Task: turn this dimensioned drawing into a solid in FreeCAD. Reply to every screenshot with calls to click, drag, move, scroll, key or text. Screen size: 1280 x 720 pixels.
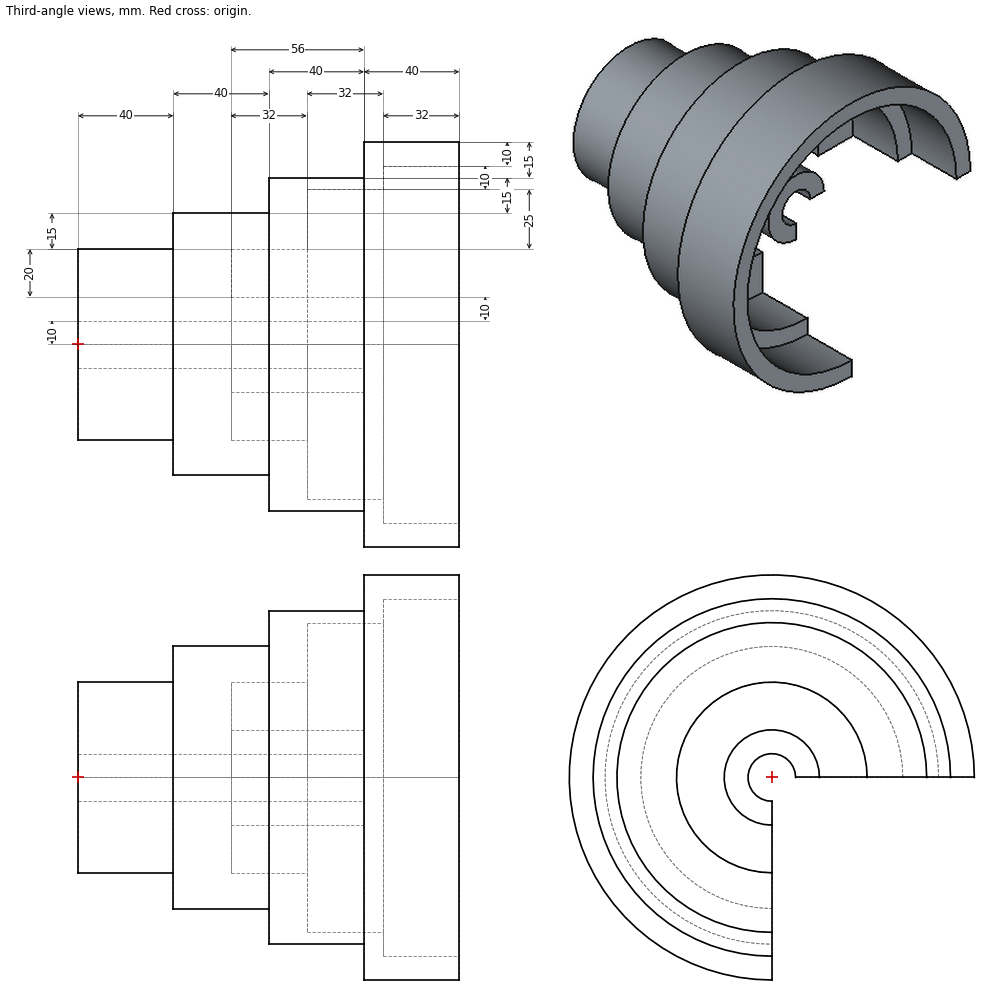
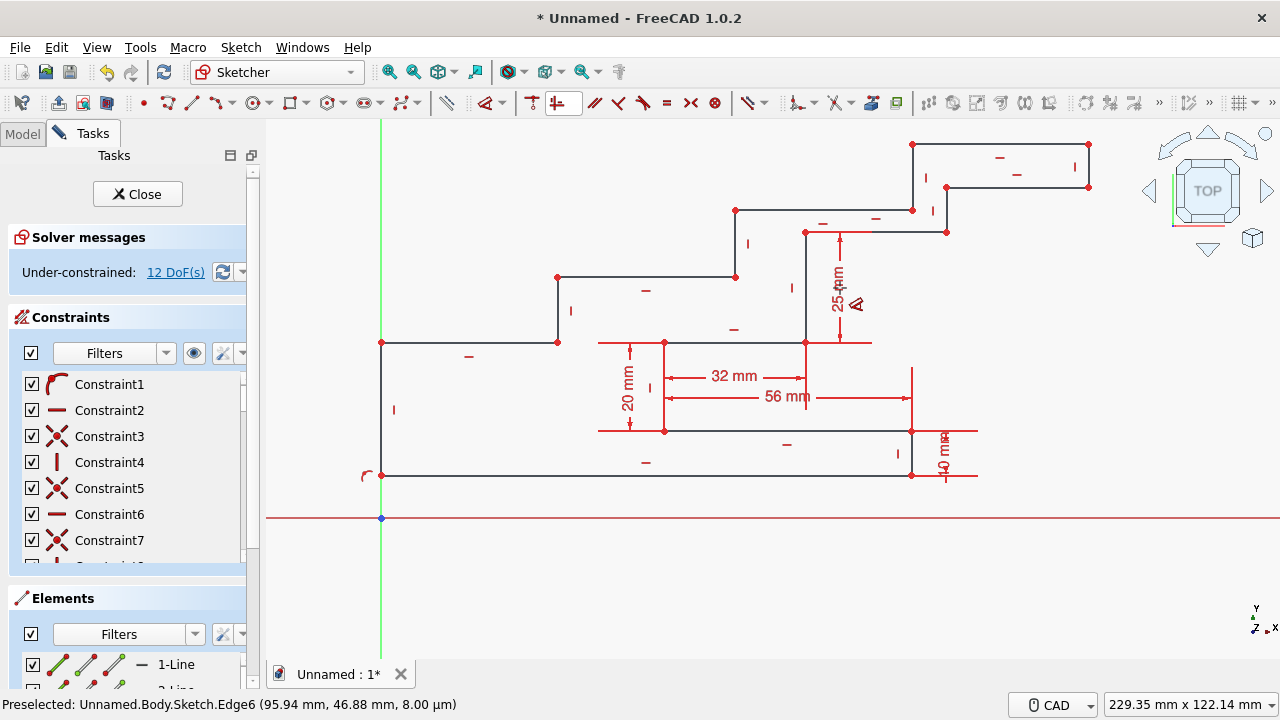
click(848, 232)
click(926, 198)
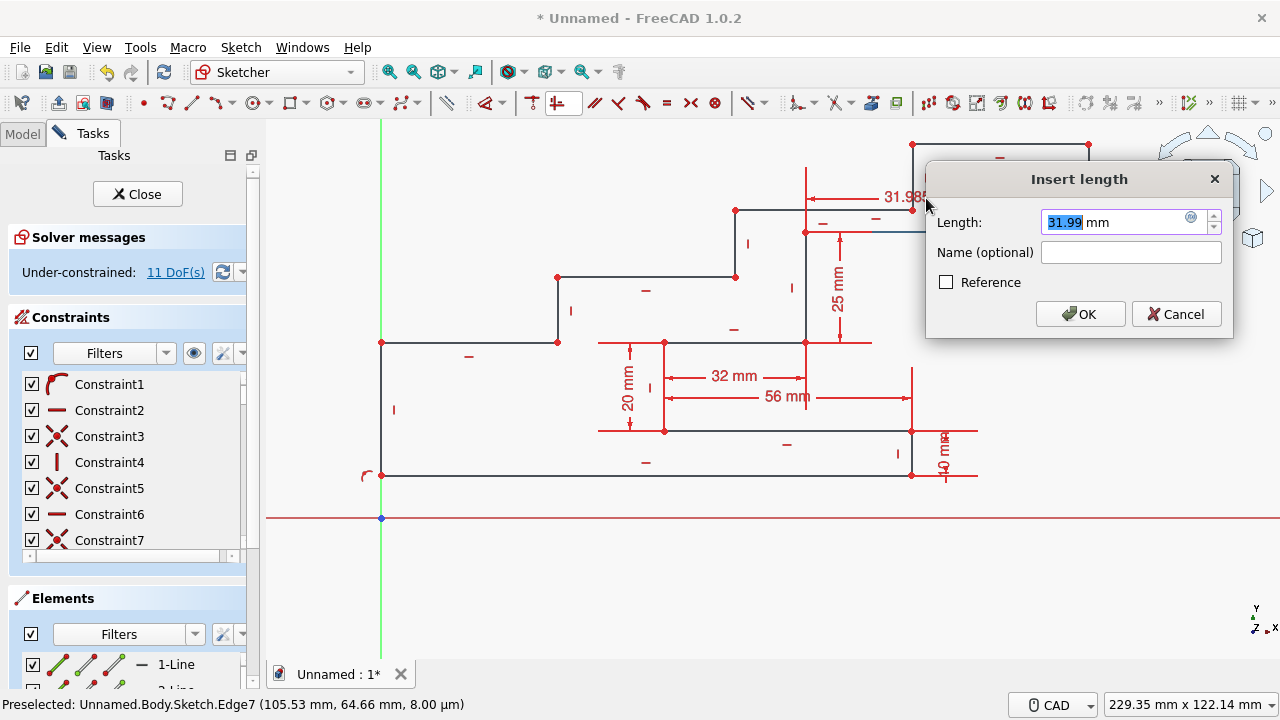
text(32)
key(Return)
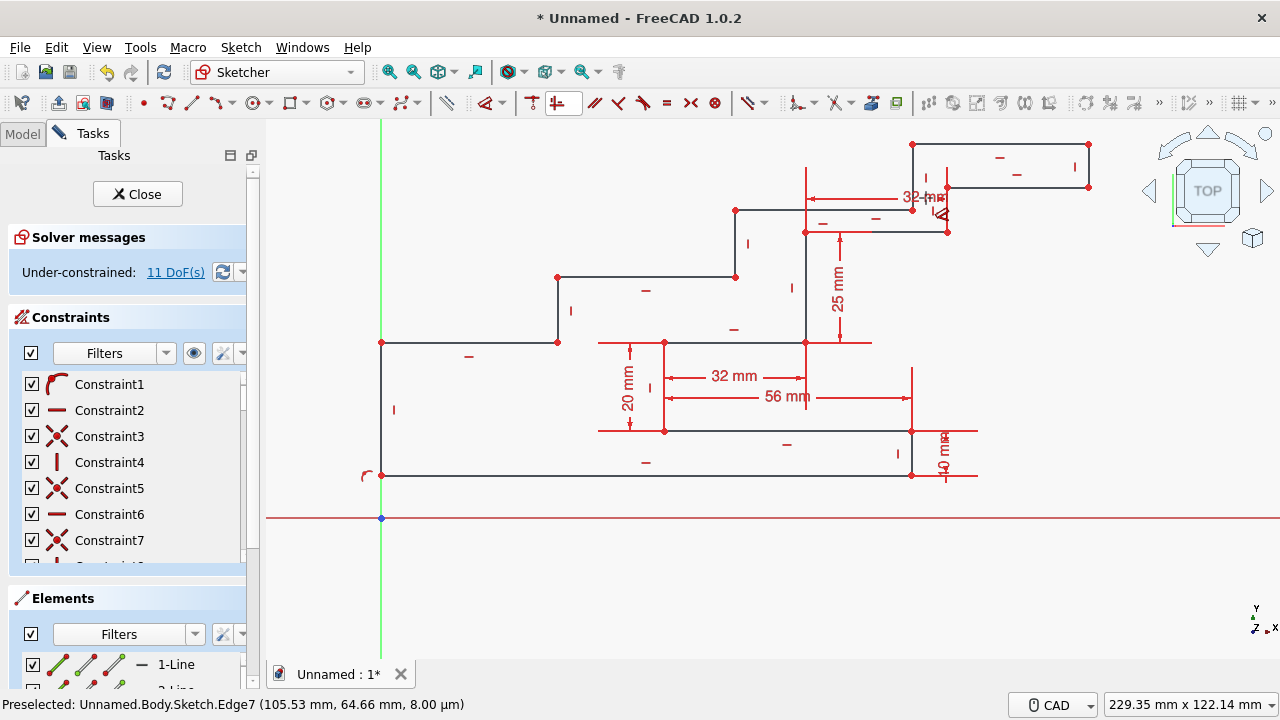
click(947, 219)
click(981, 220)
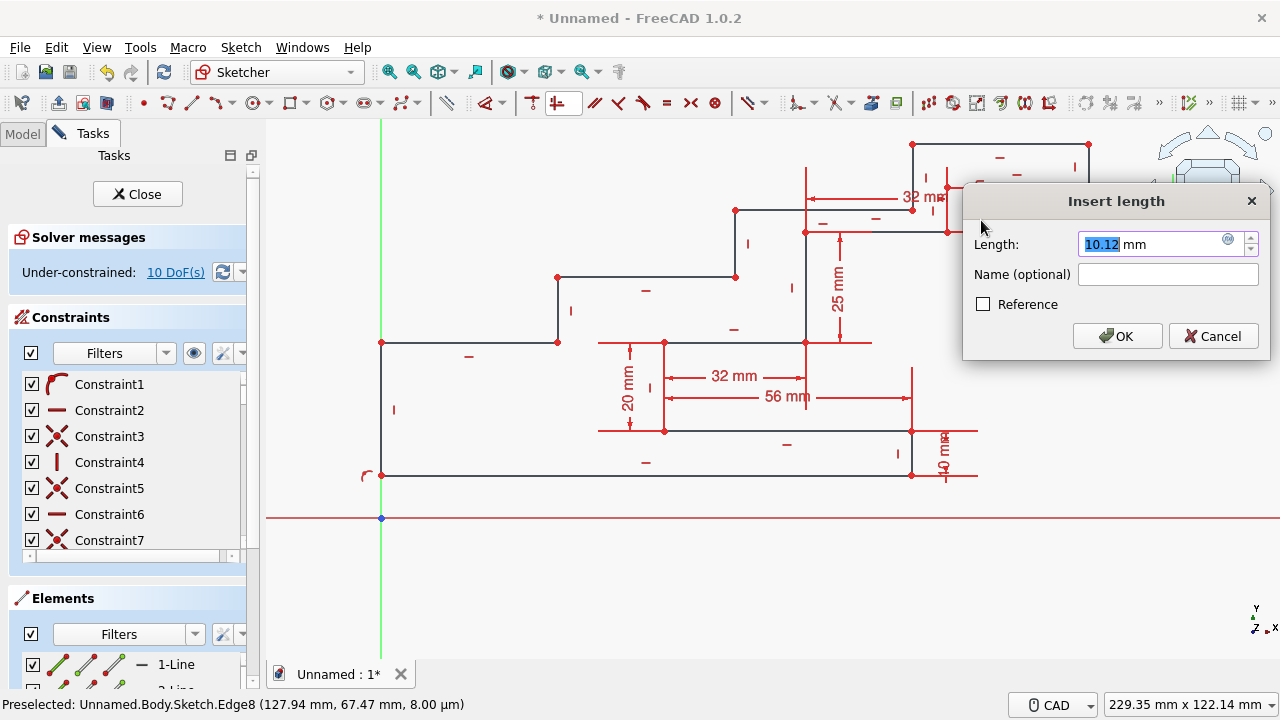
text(10)
key(Return)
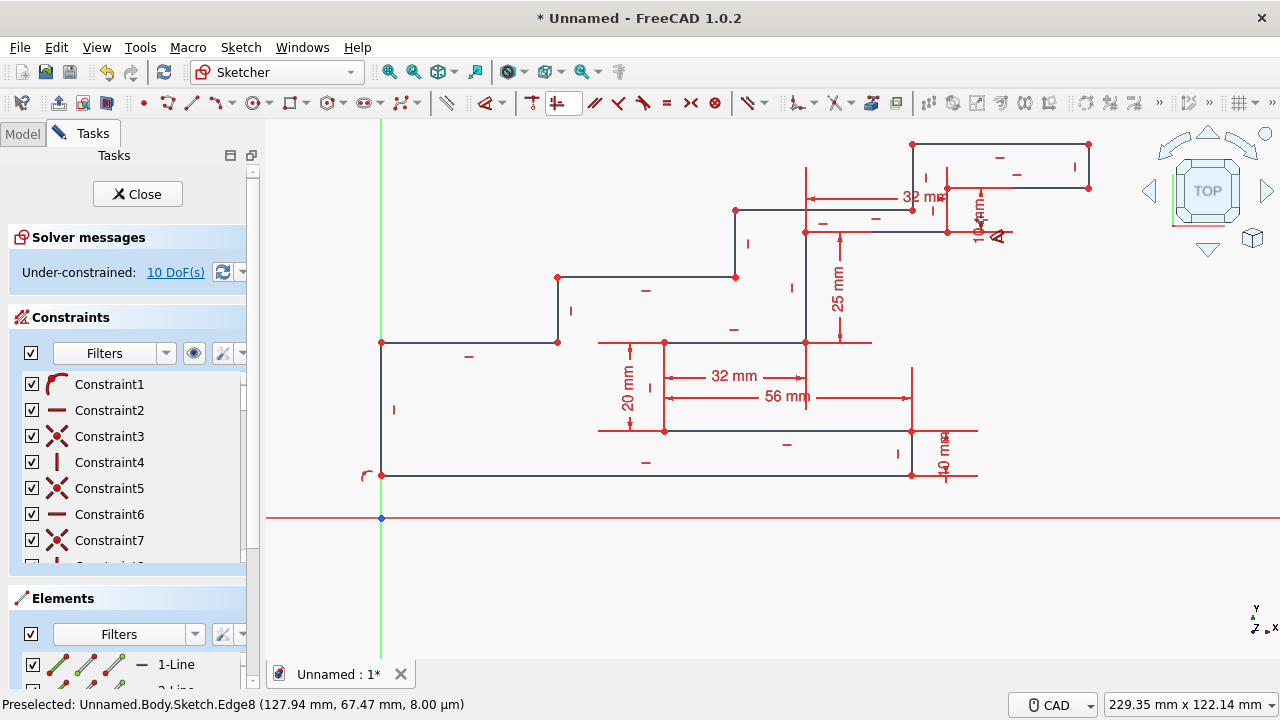
click(990, 188)
click(1067, 222)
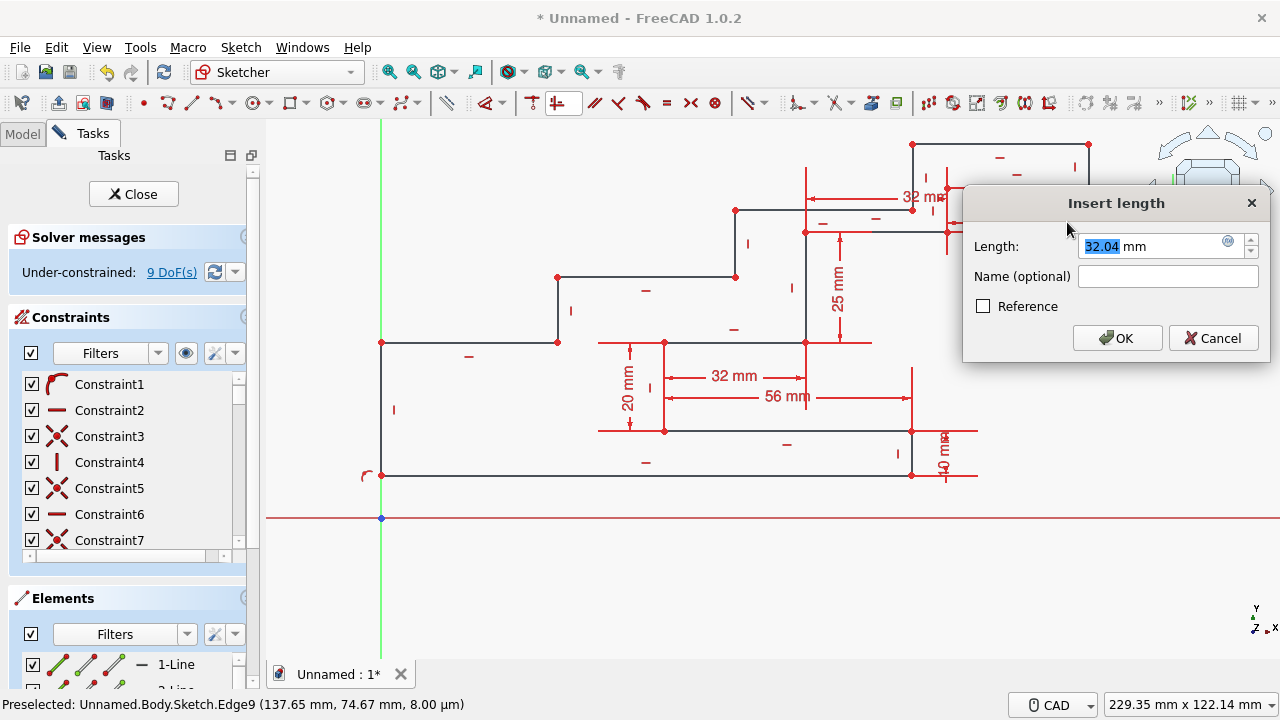
text(32)
key(Return)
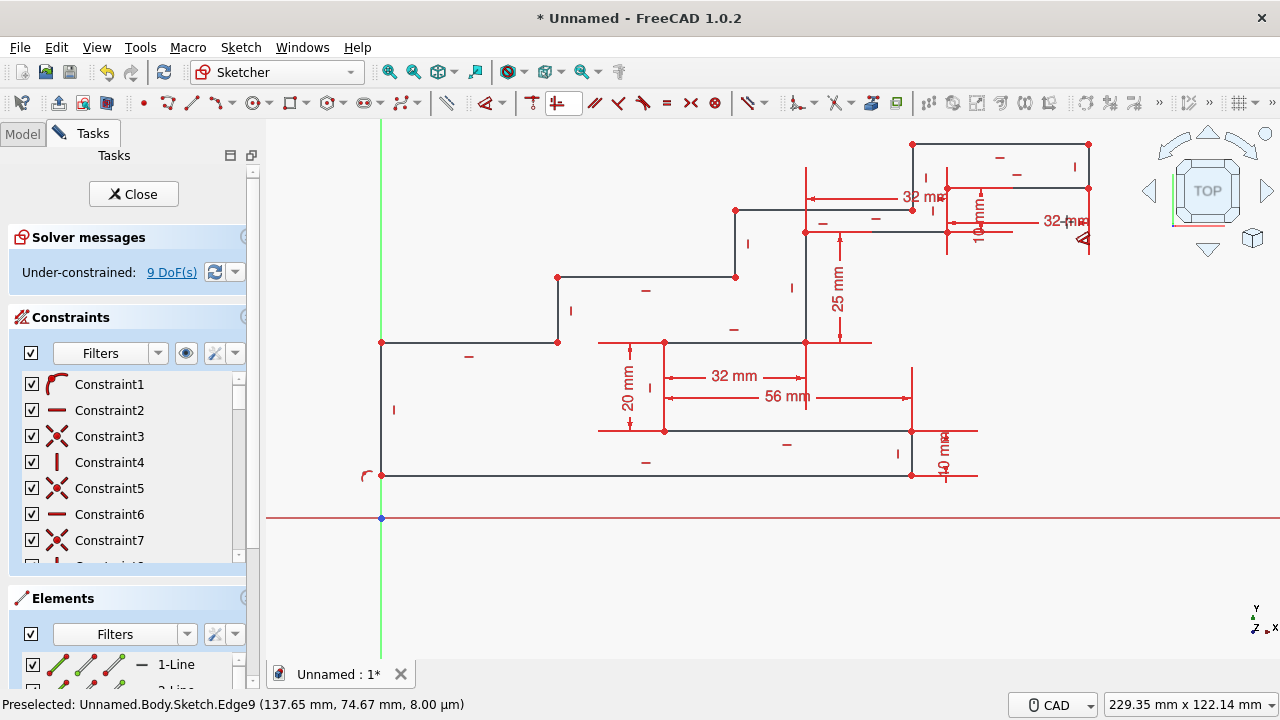
click(1089, 175)
click(1055, 168)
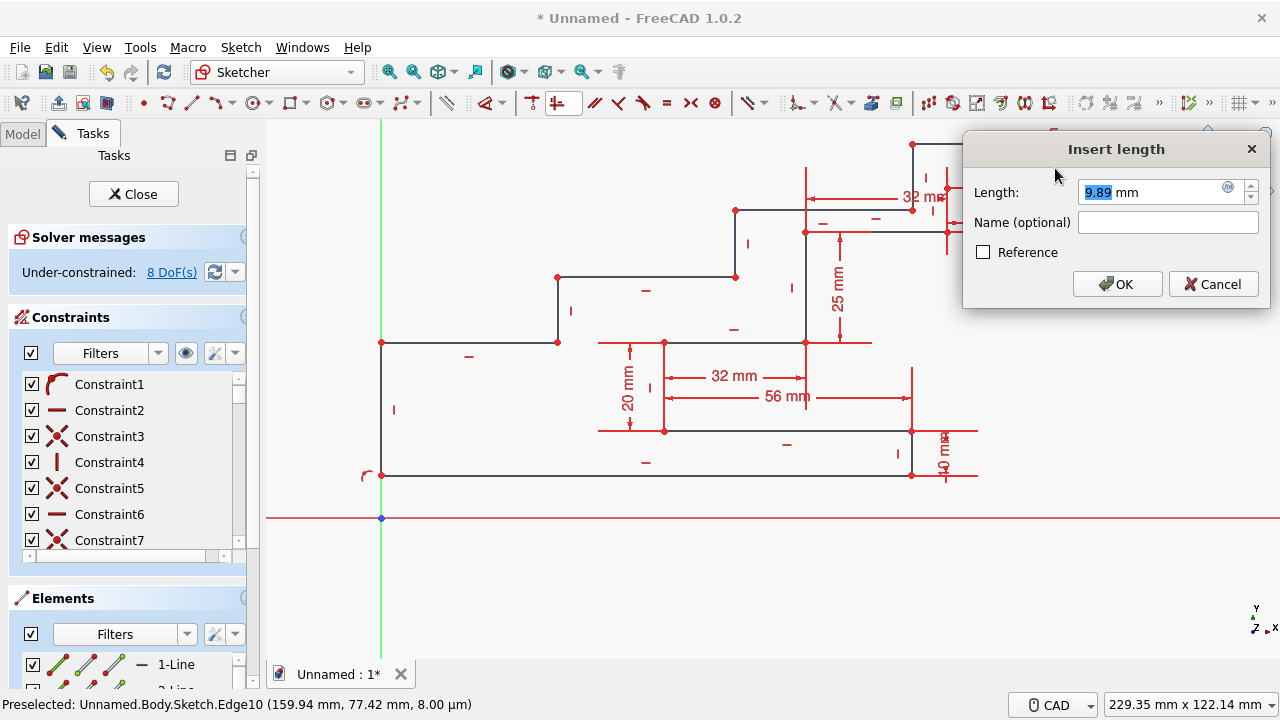
text(10)
key(Return)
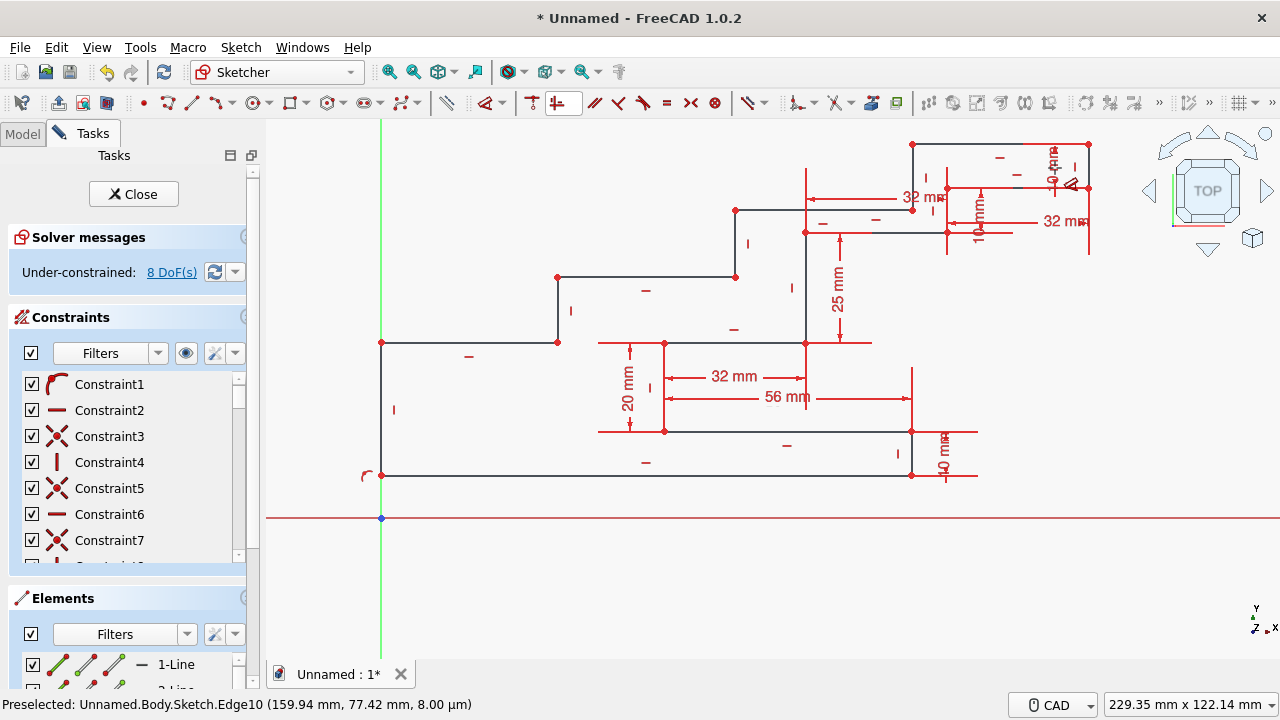
scroll(566, 631, down, 1)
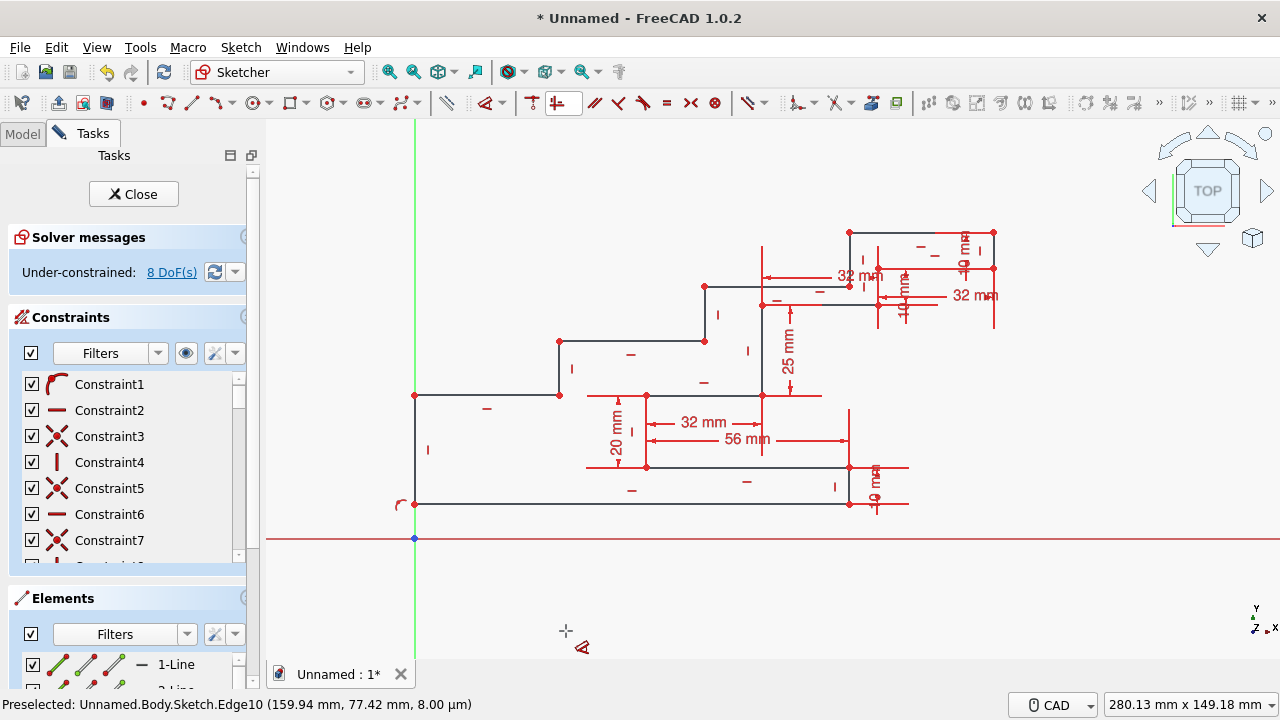
click(951, 233)
click(922, 199)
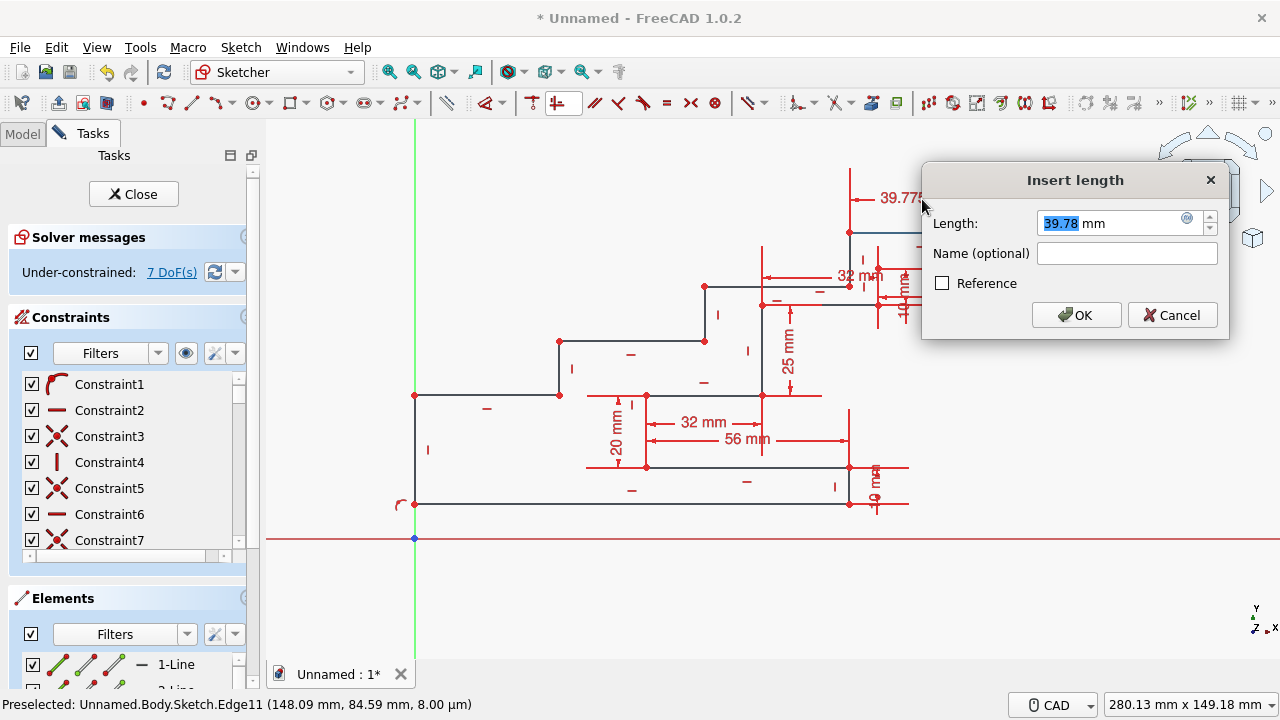
text(40)
key(Return)